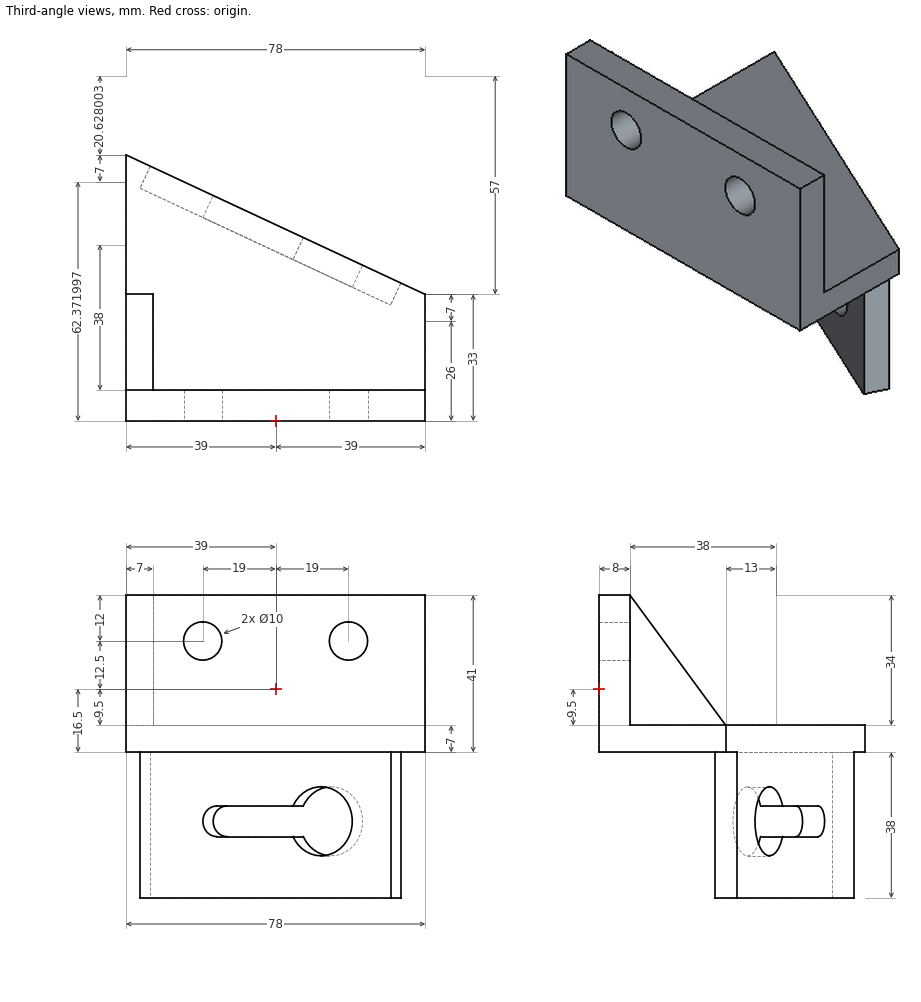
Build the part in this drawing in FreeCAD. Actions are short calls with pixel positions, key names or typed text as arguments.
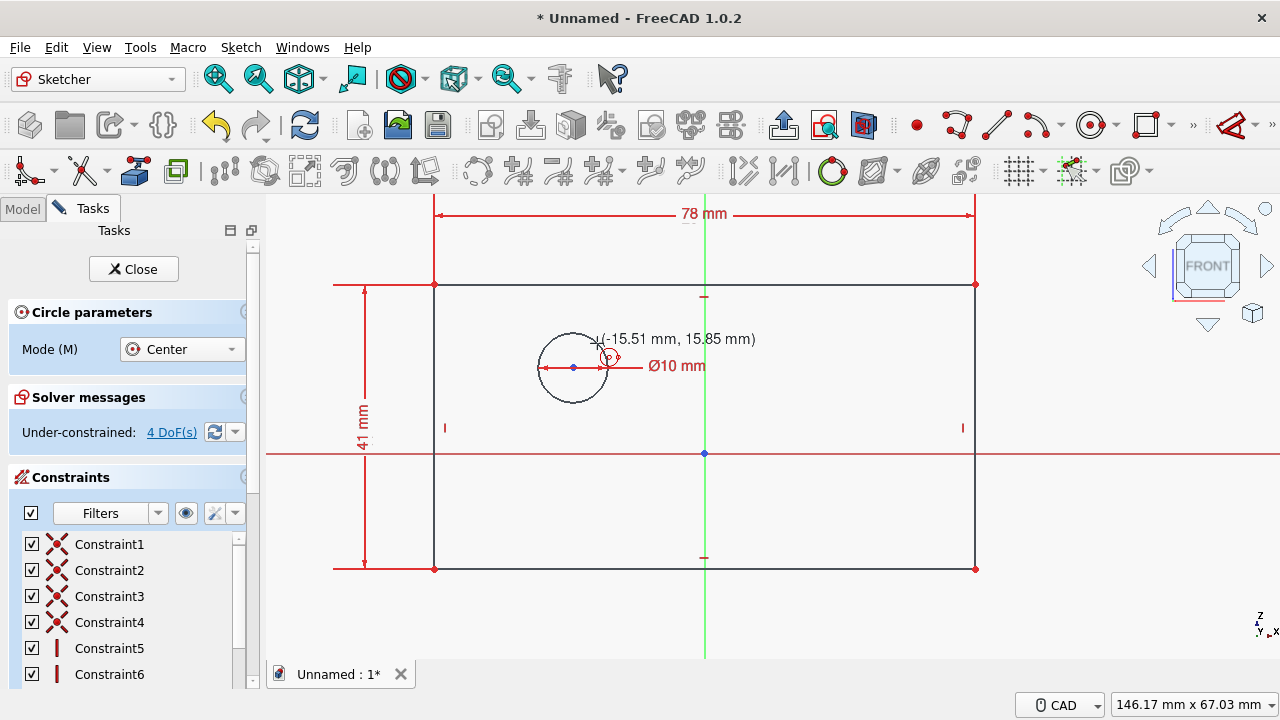
click(836, 367)
move(861, 343)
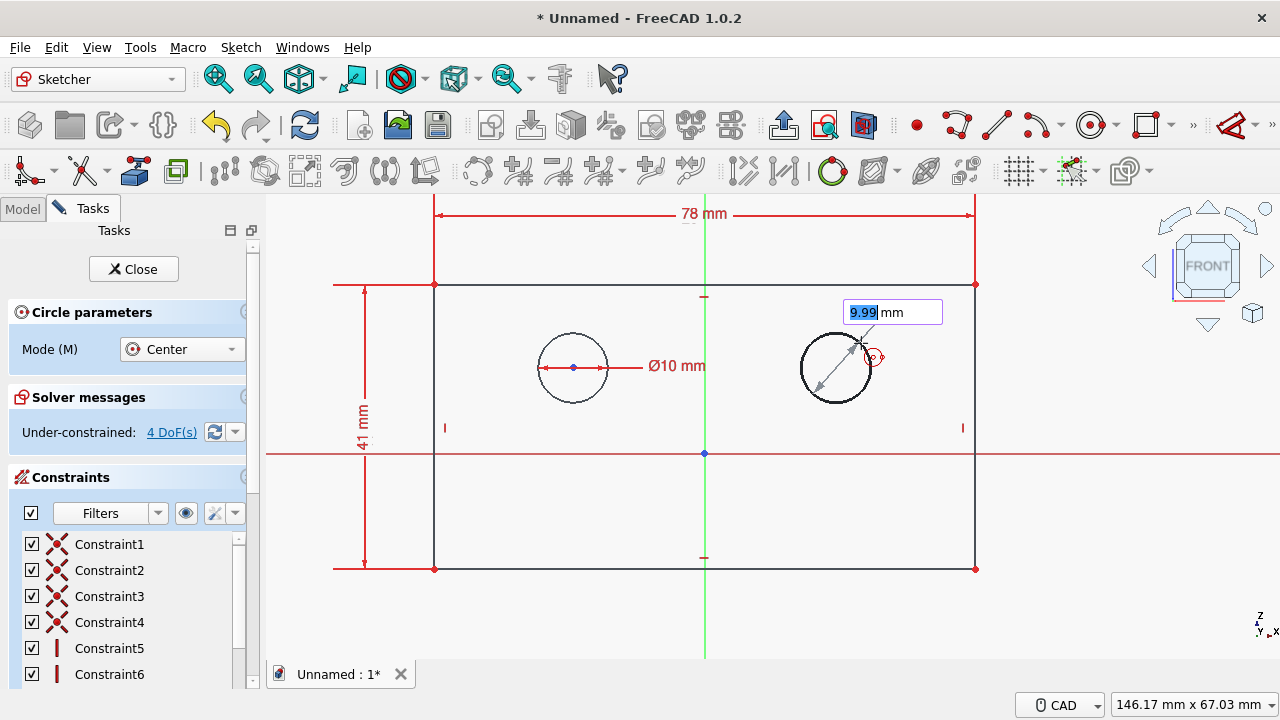
text(10)
key(Return)
key(Escape)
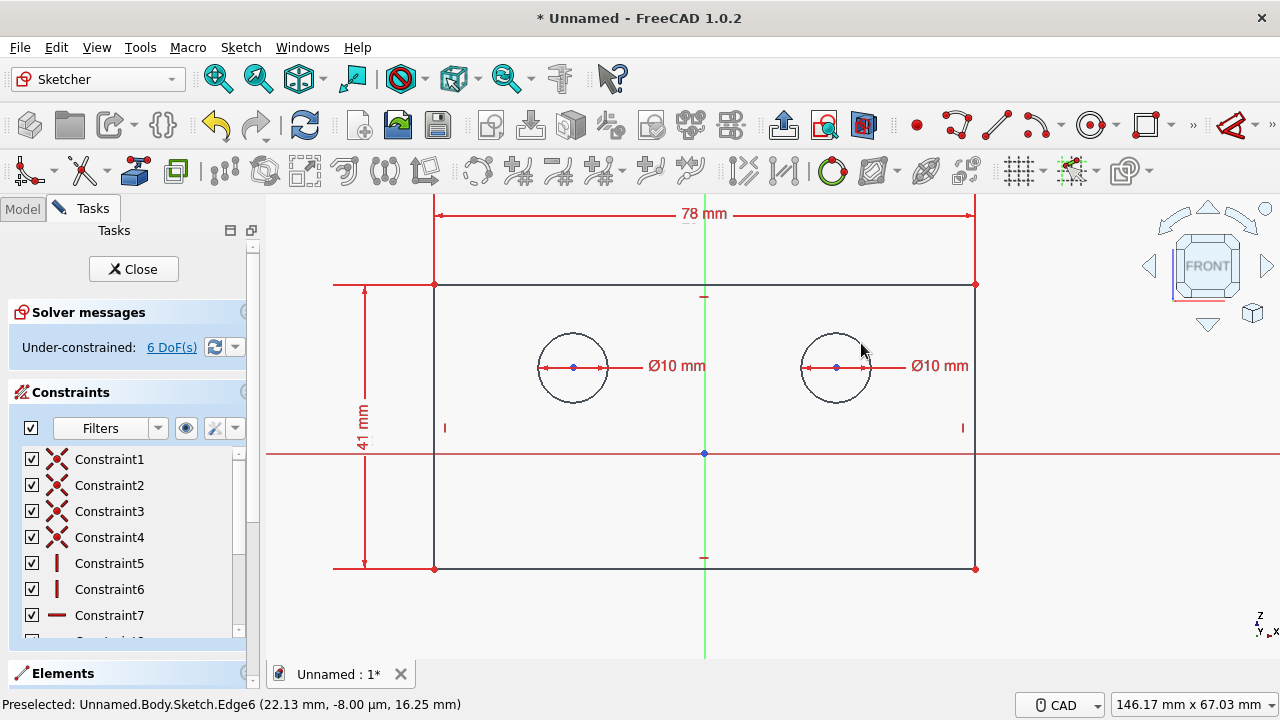
click(573, 368)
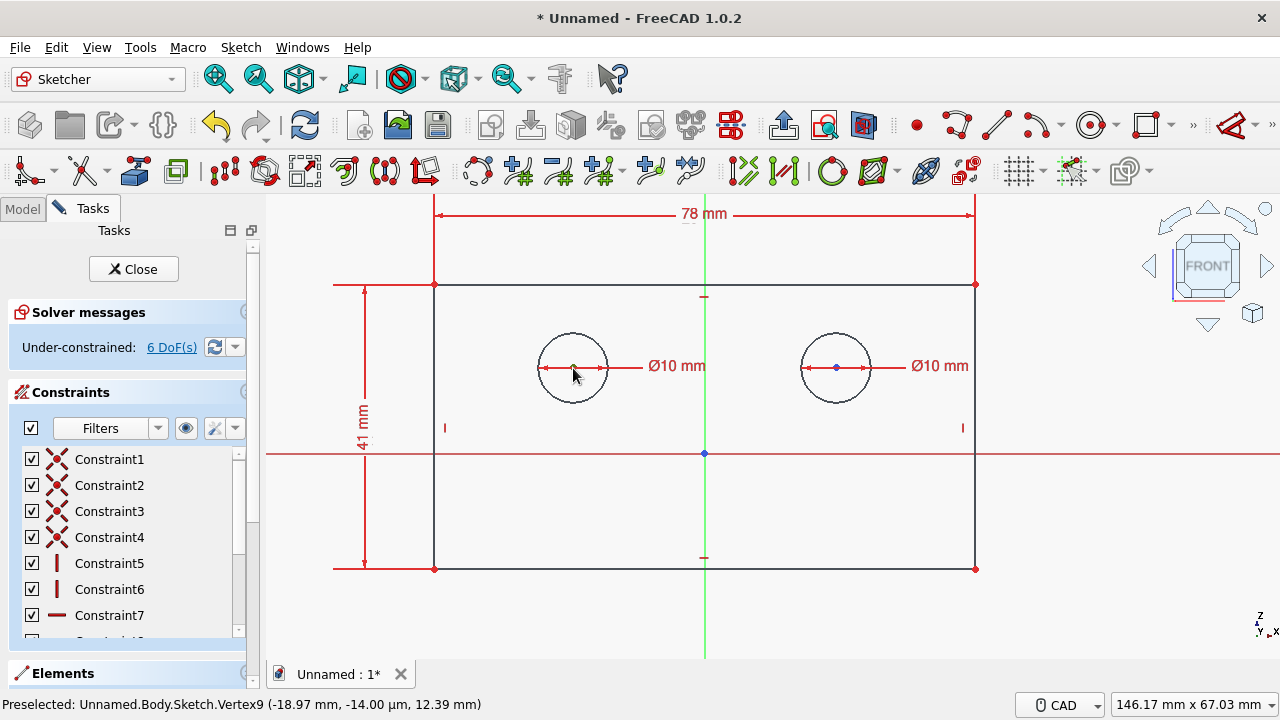
click(836, 368)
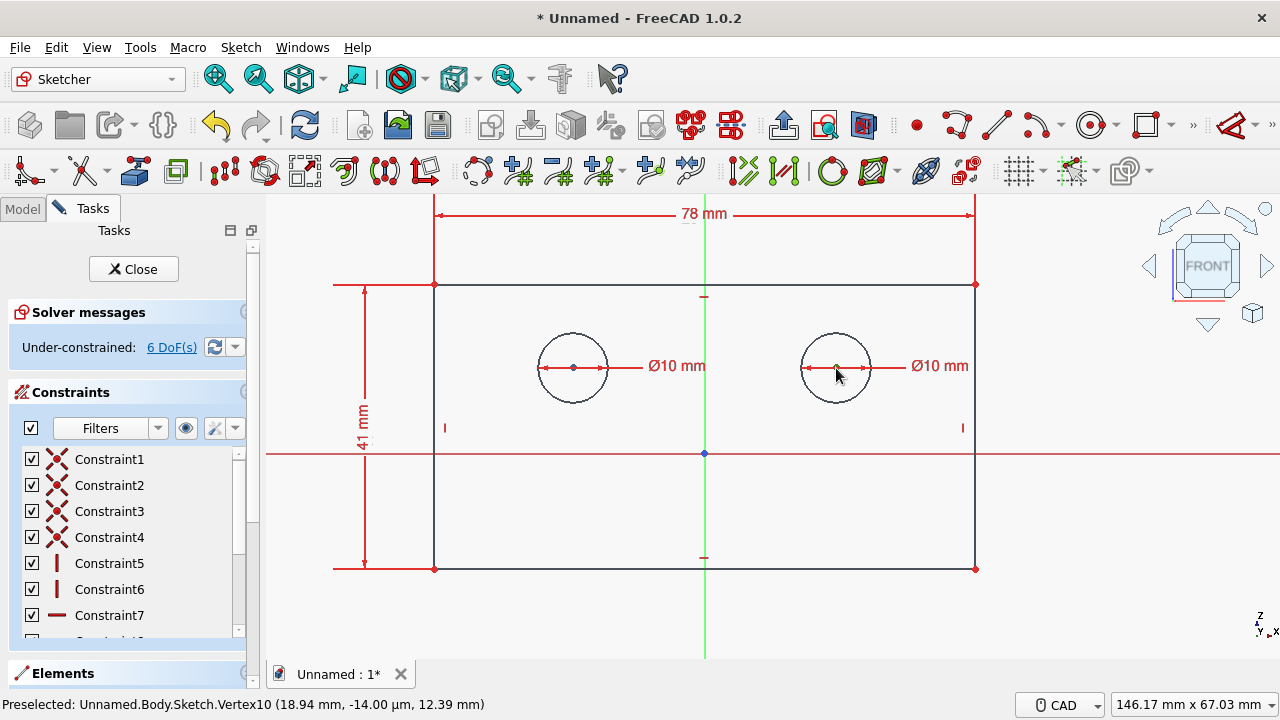
key(h)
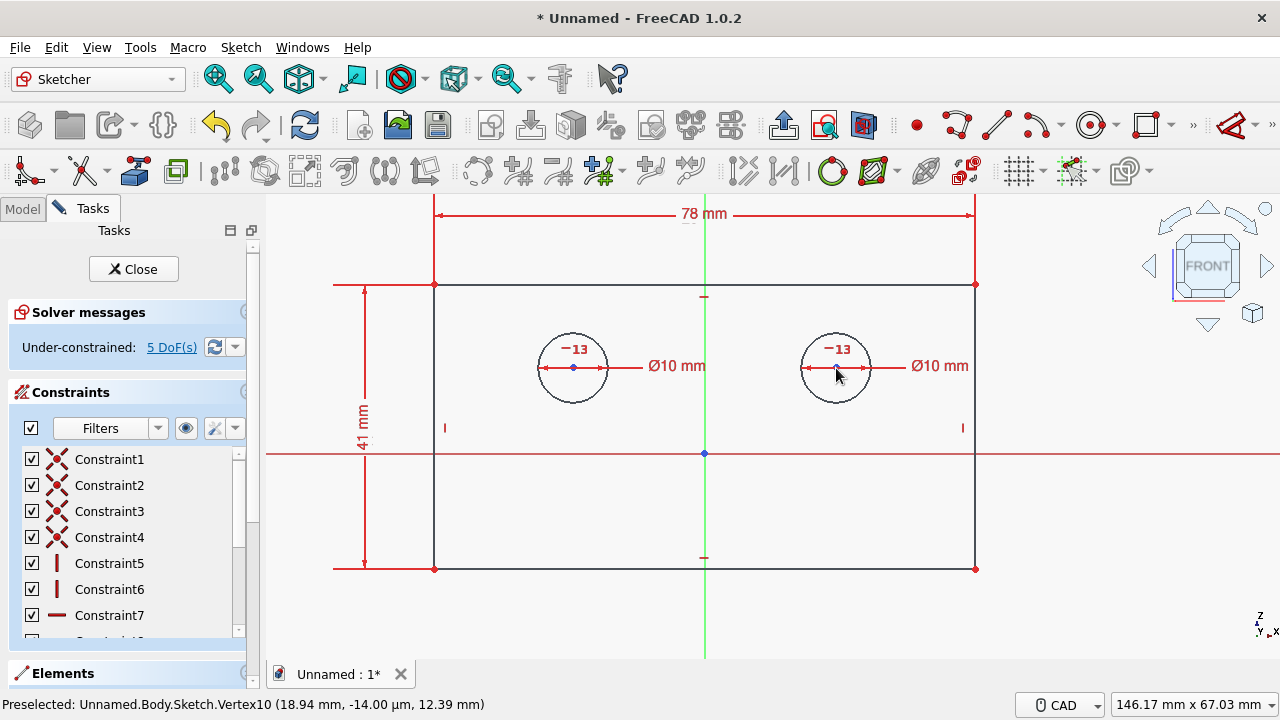
click(1232, 126)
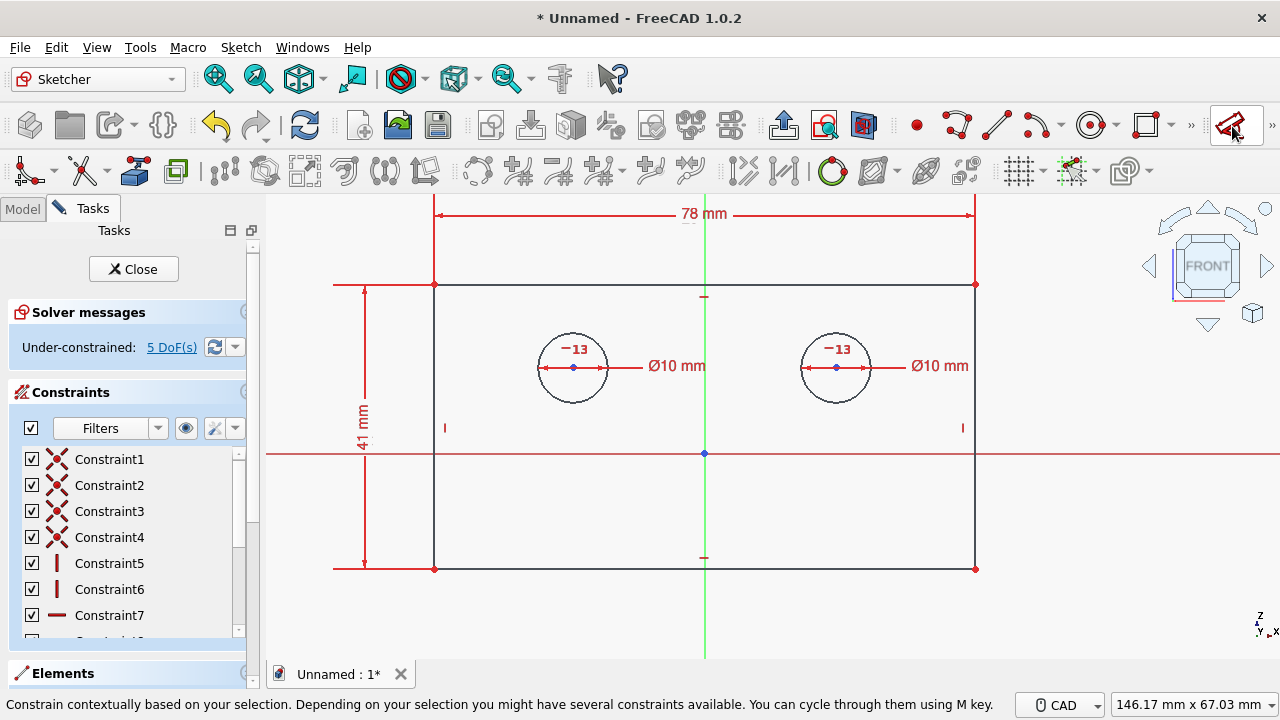
click(573, 368)
click(639, 334)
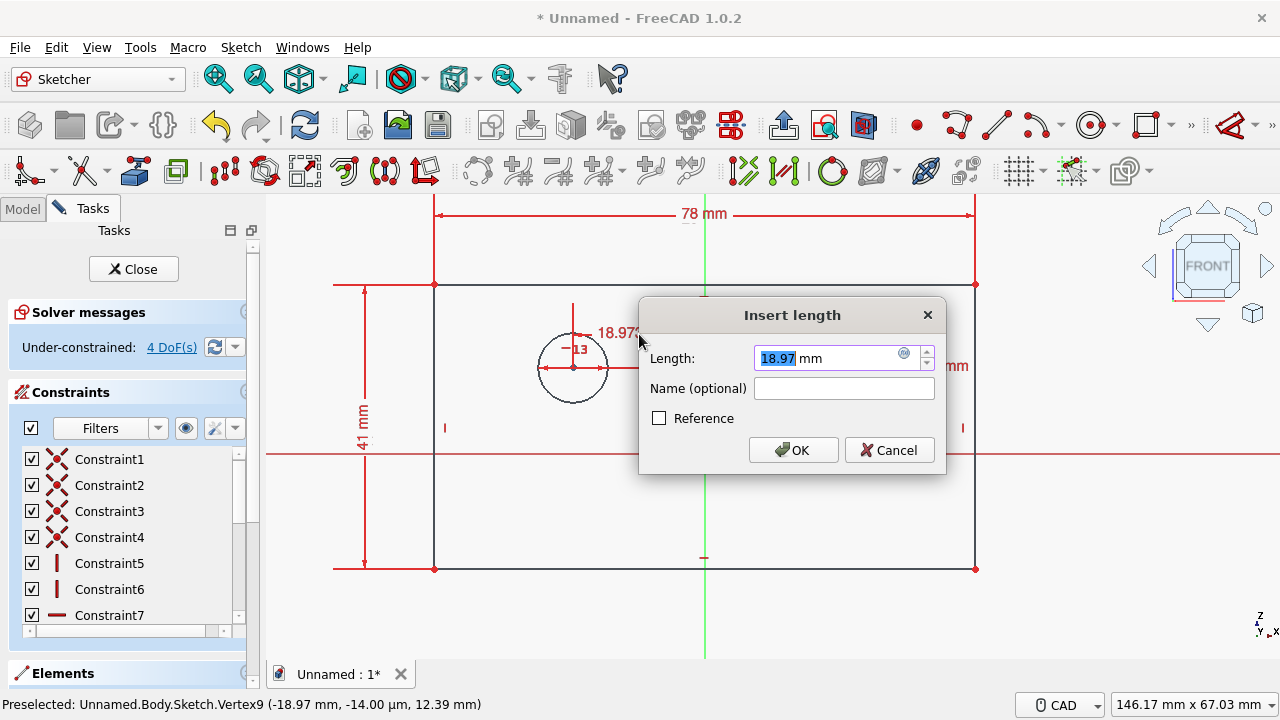
text(19)
key(Return)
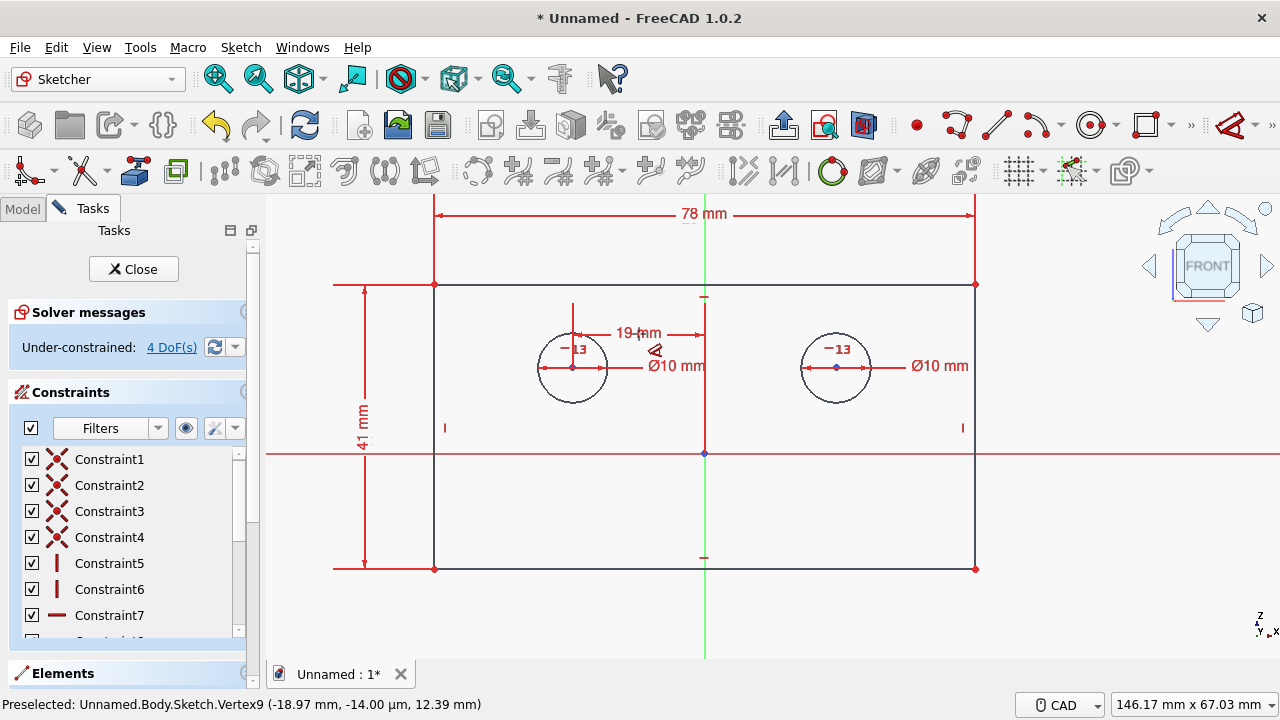
click(836, 368)
click(770, 334)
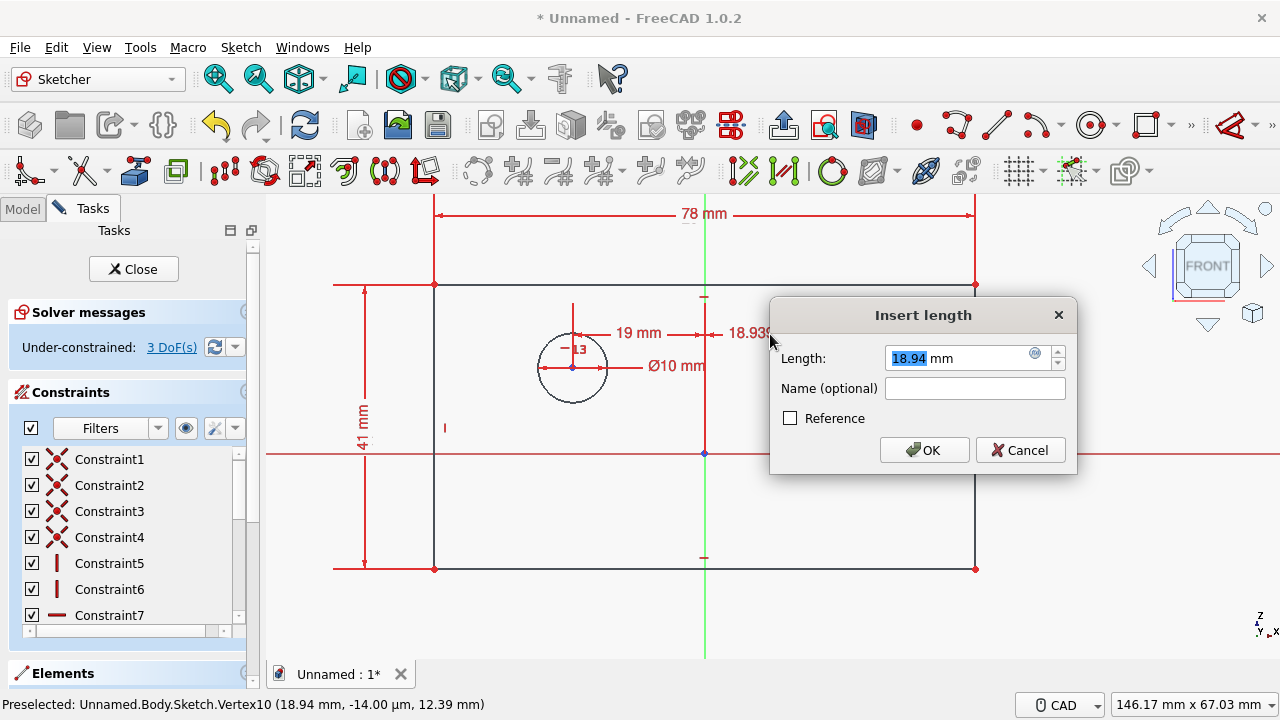
text(19)
key(Return)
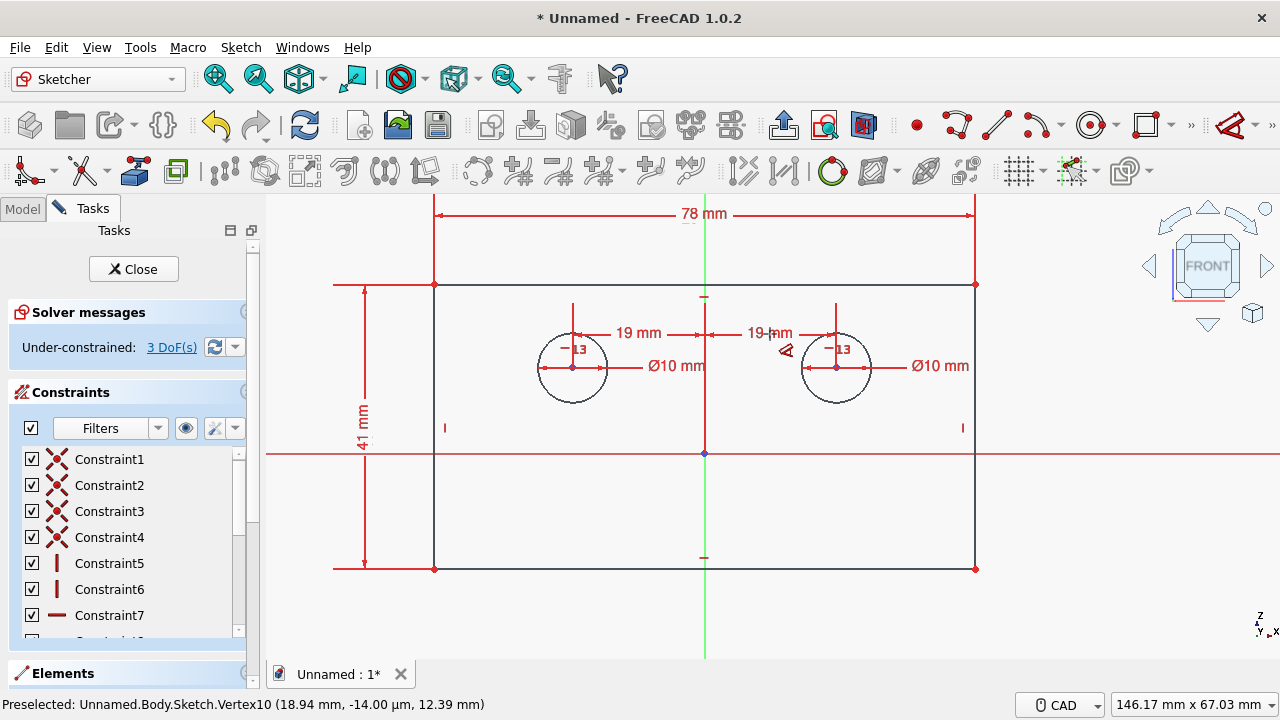
click(434, 285)
click(569, 251)